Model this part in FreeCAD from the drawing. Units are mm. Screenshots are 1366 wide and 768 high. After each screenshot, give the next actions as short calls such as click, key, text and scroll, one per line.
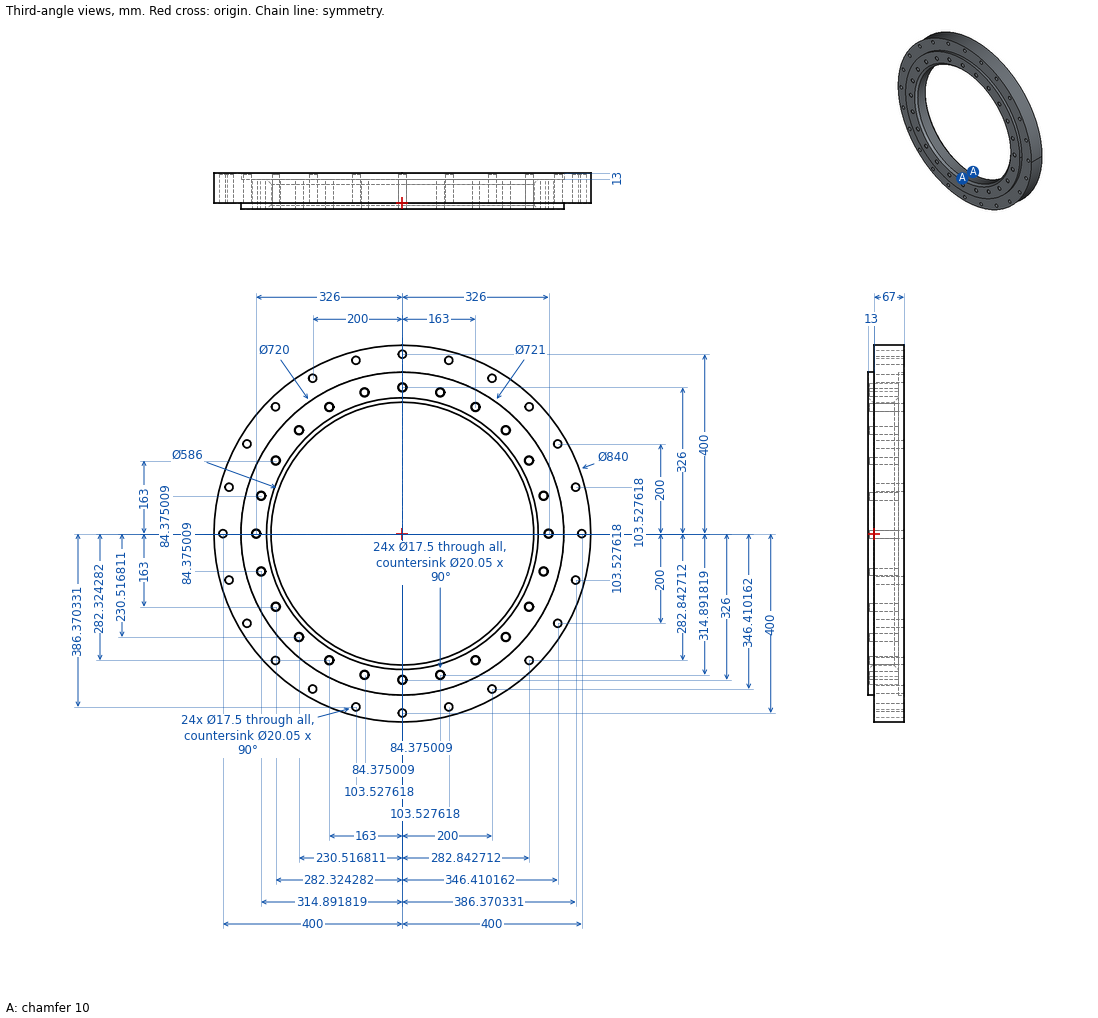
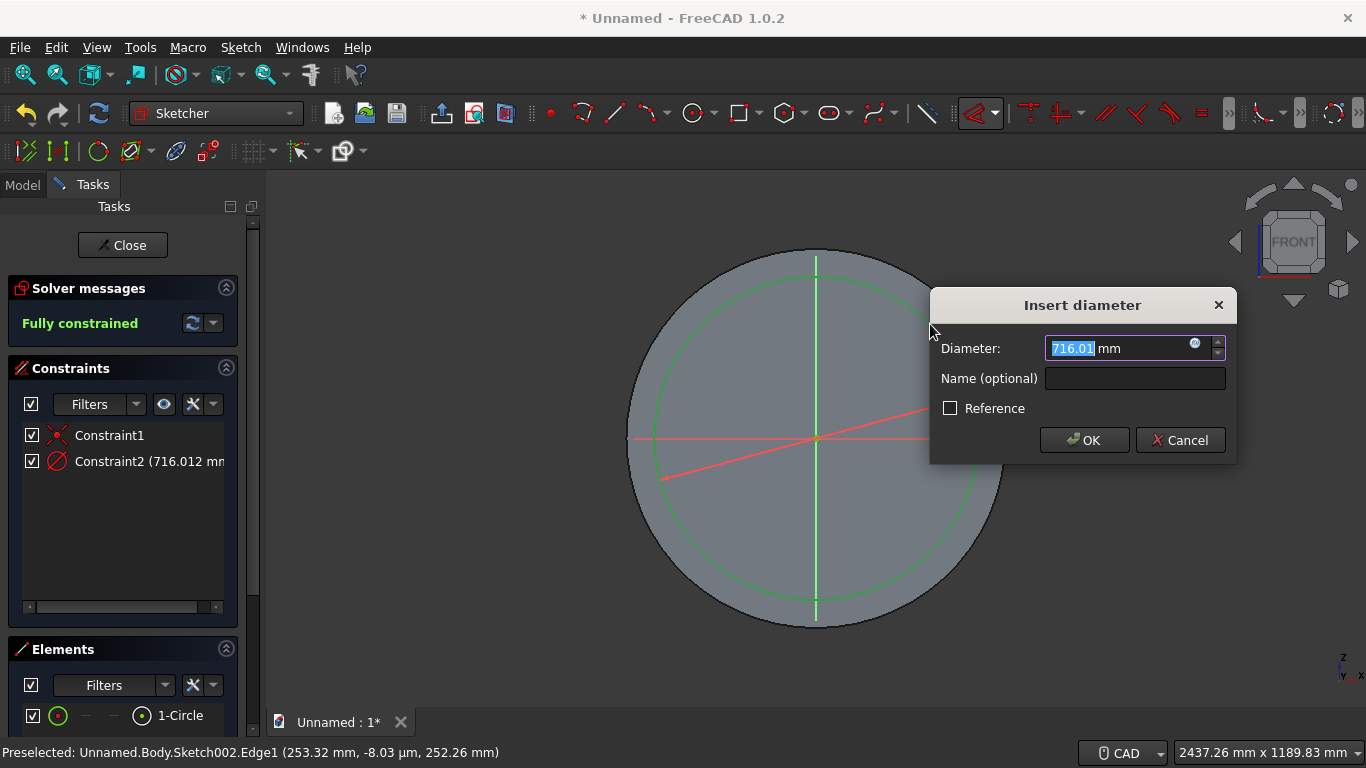
text(720)
key(Return)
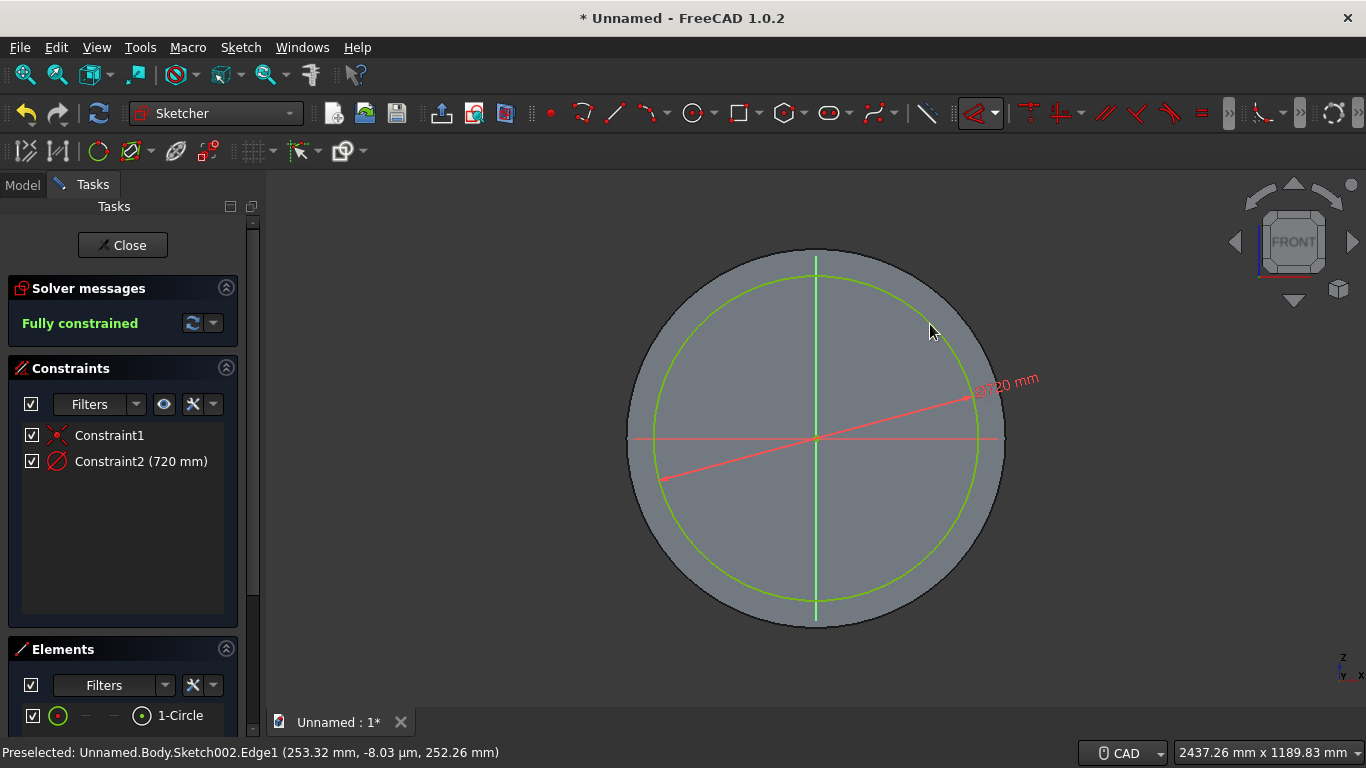
click(123, 245)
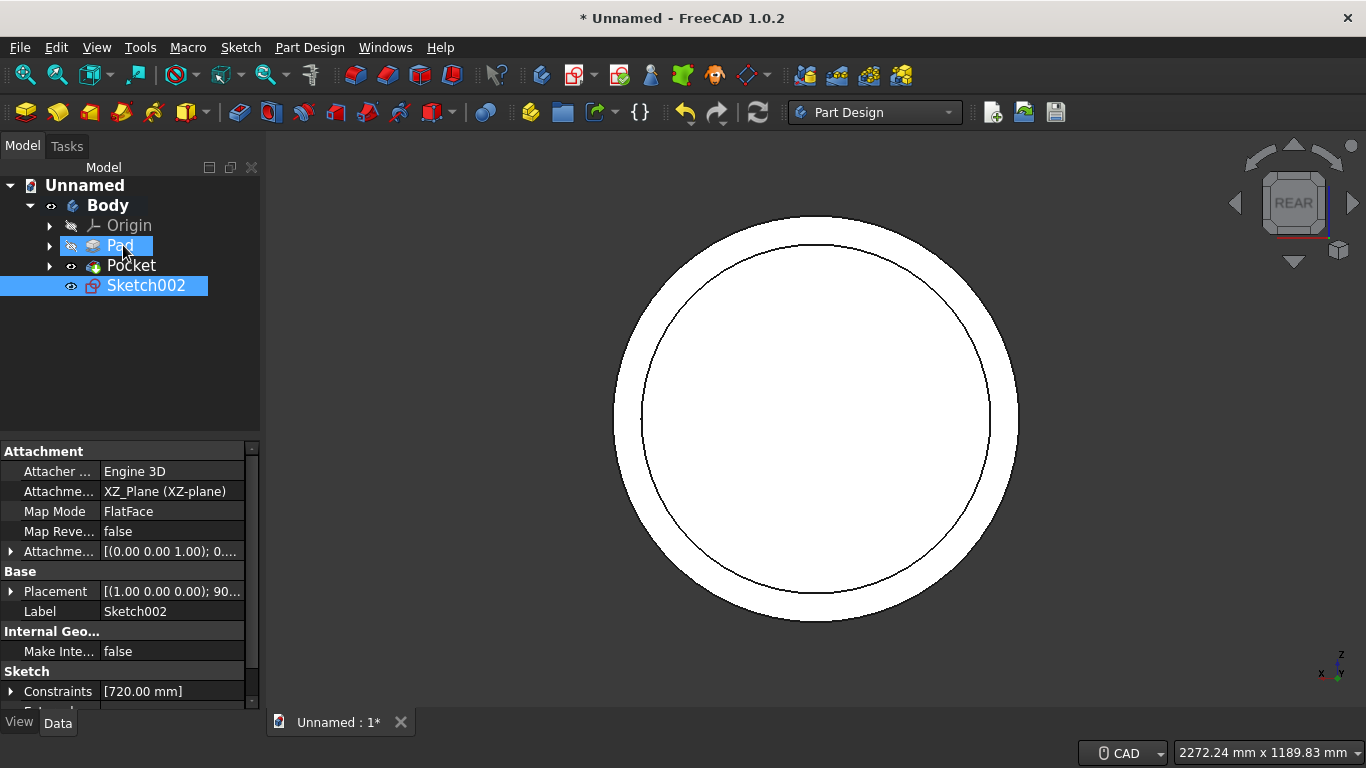
click(26, 112)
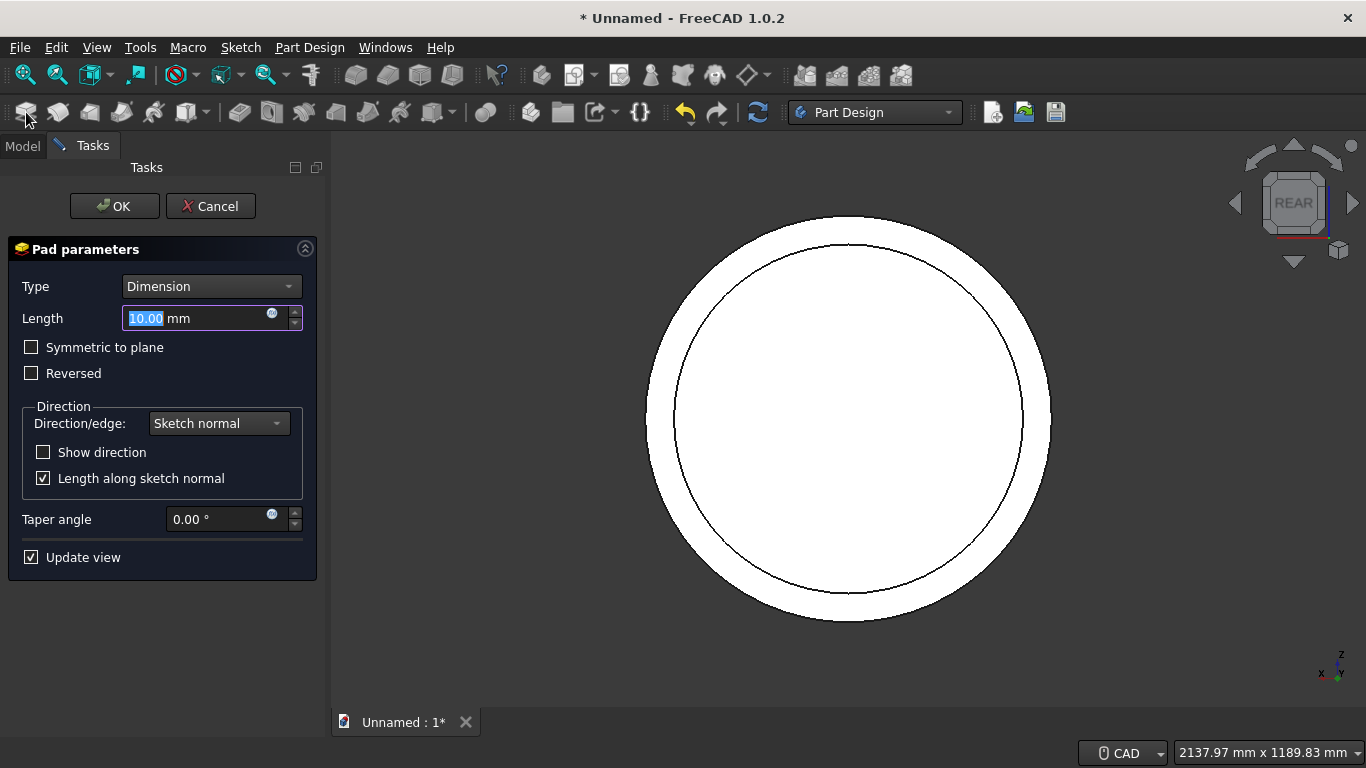
text(13)
key(Tab)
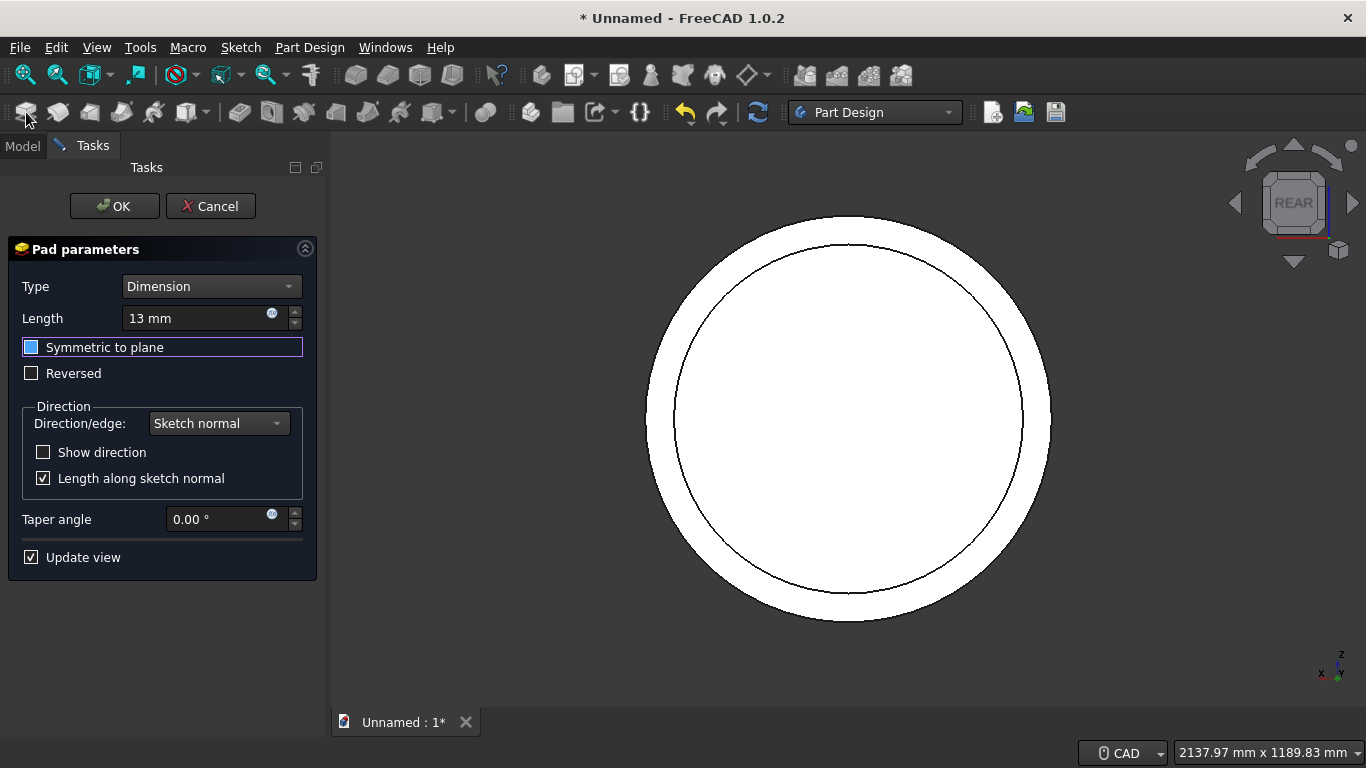
click(115, 206)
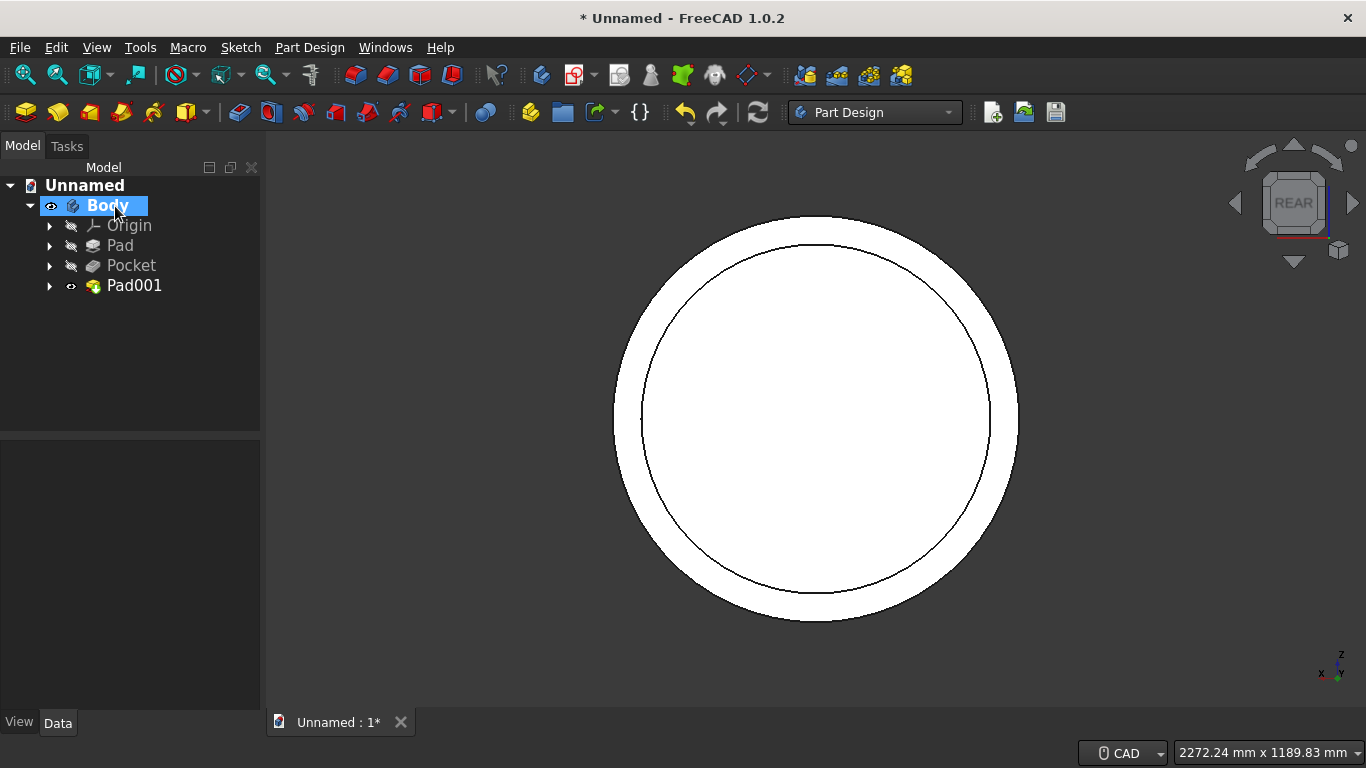
click(990, 360)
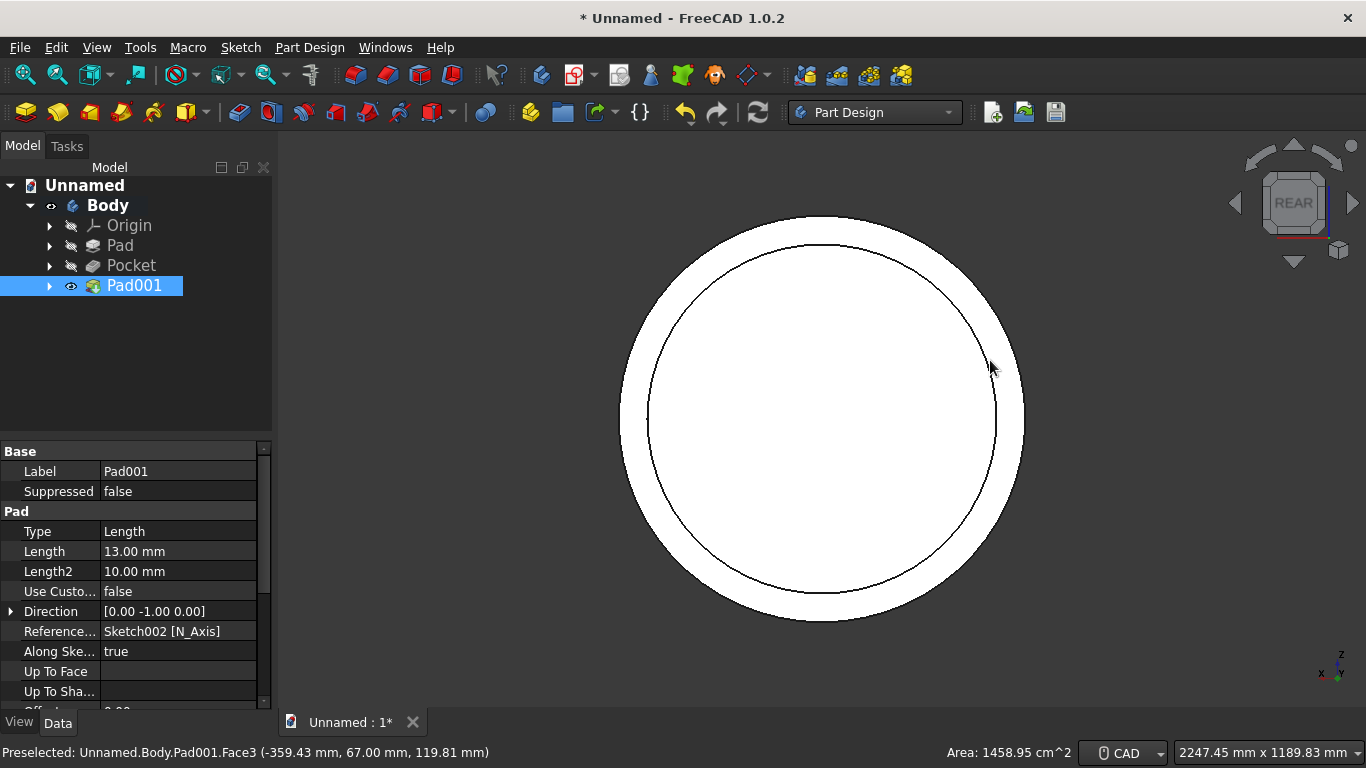
click(574, 76)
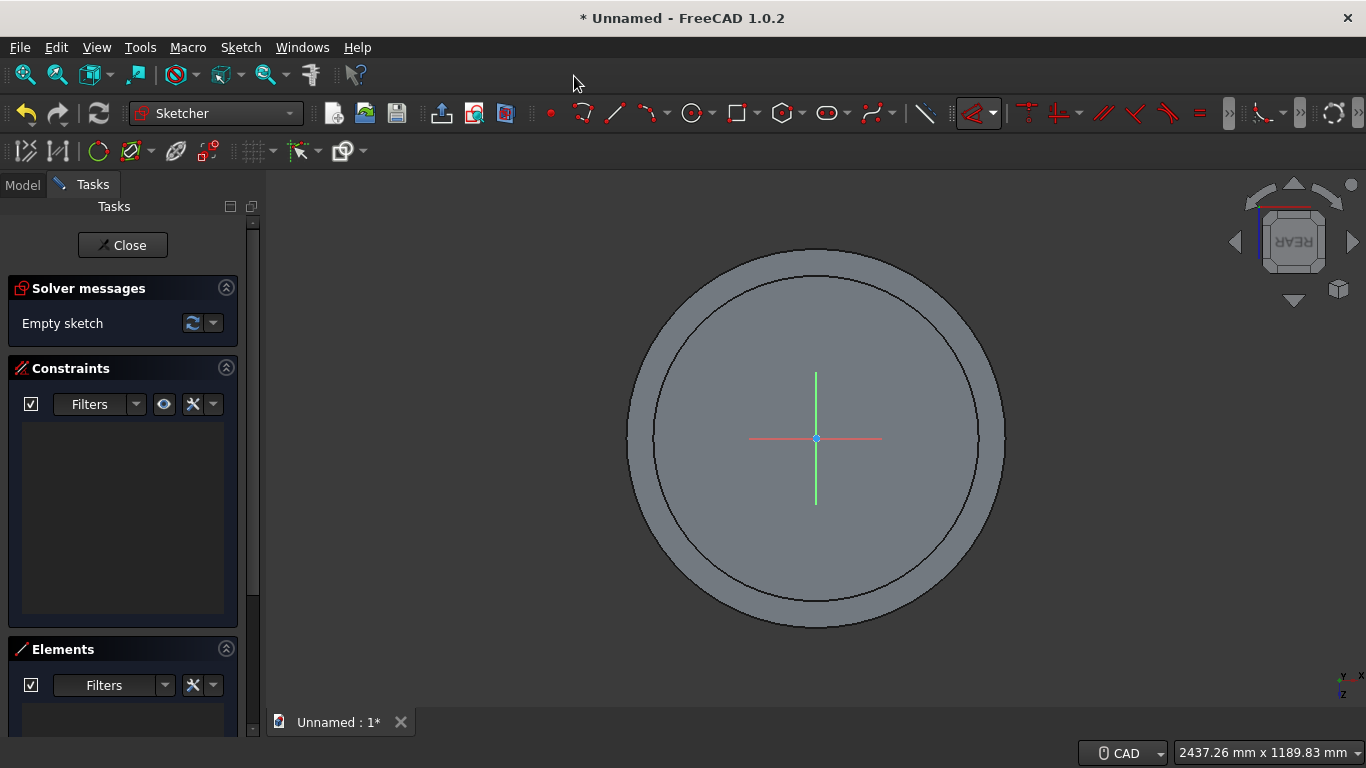
key(g)
key(c)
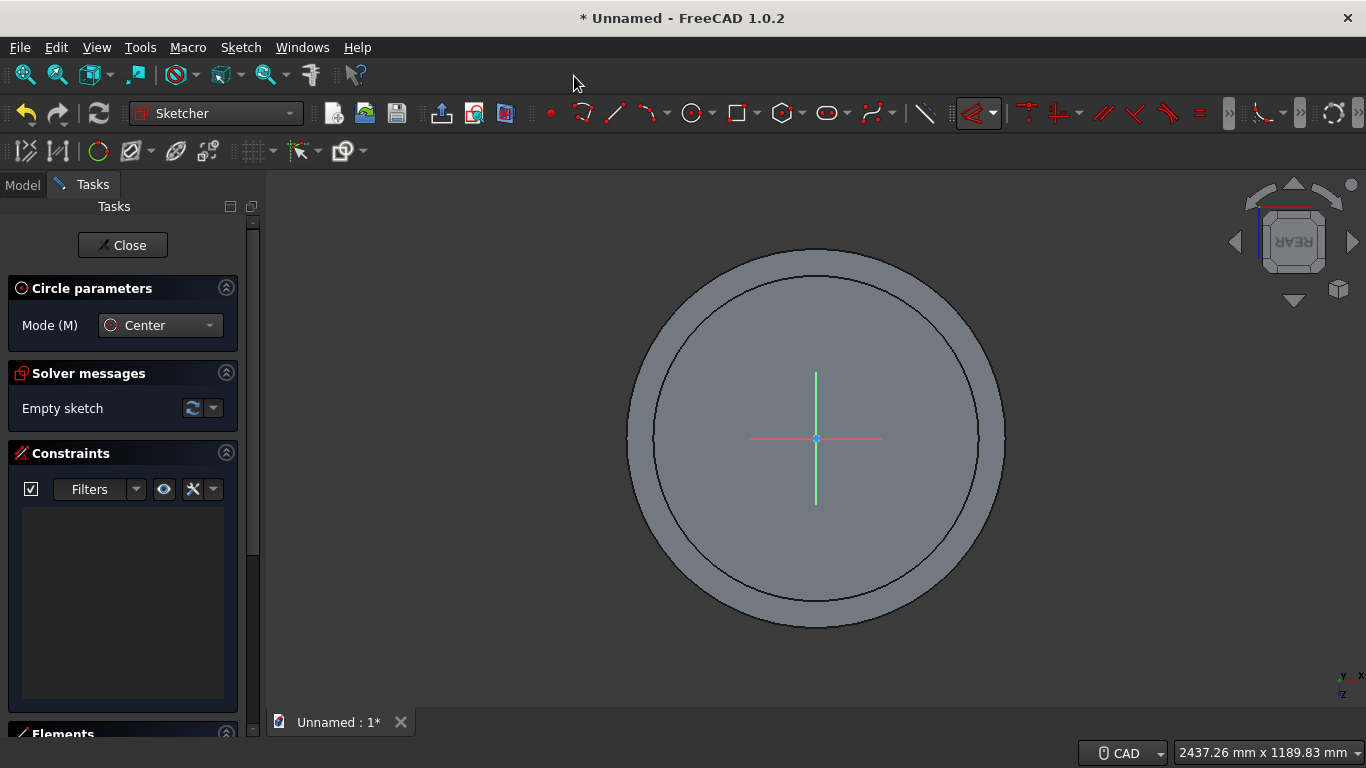
scroll(769, 264, up, 9)